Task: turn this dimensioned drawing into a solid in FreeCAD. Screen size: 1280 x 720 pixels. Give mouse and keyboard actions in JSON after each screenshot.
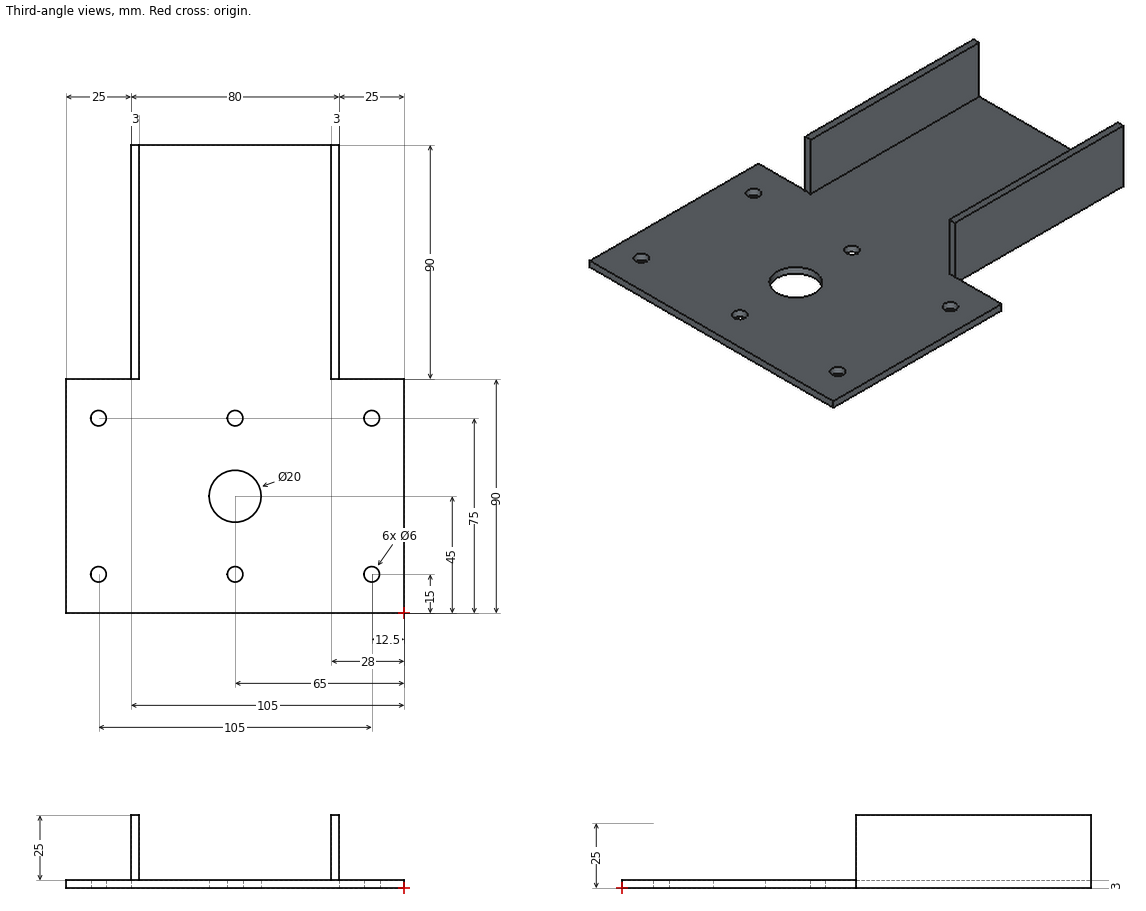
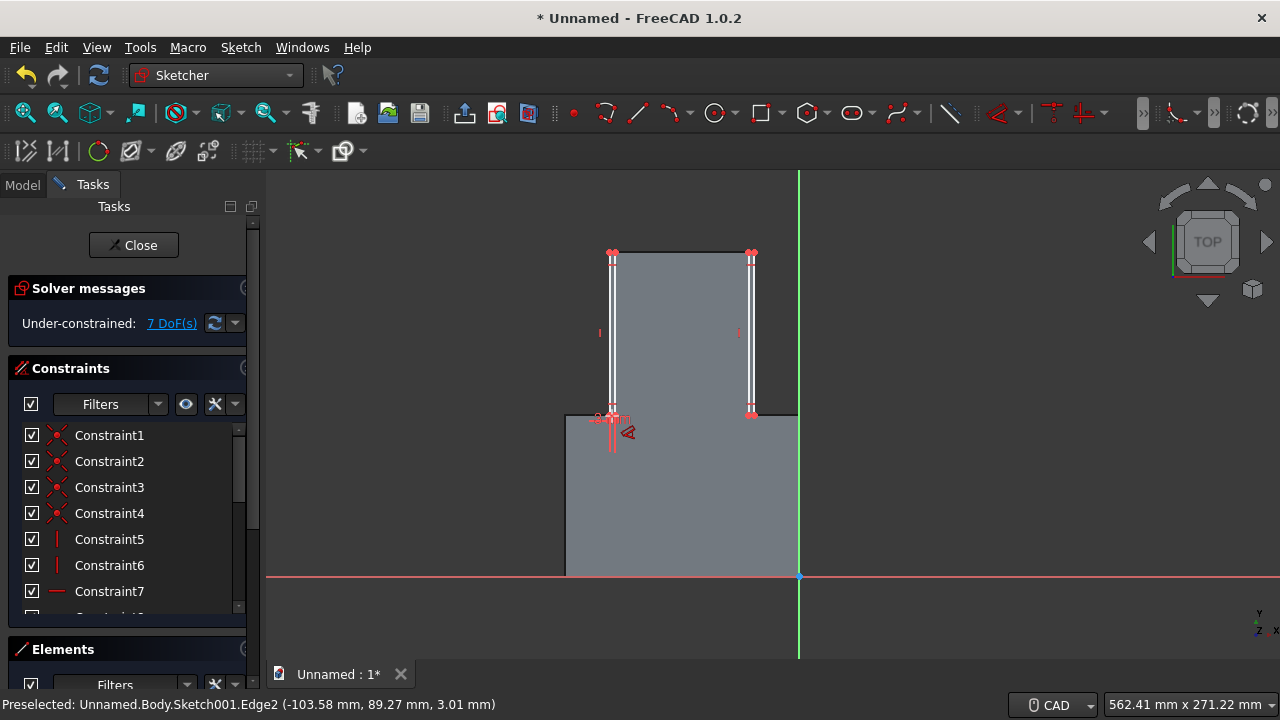
{"action": "scroll", "coordinate": [750, 416], "scroll_direction": "up", "scroll_amount": 11}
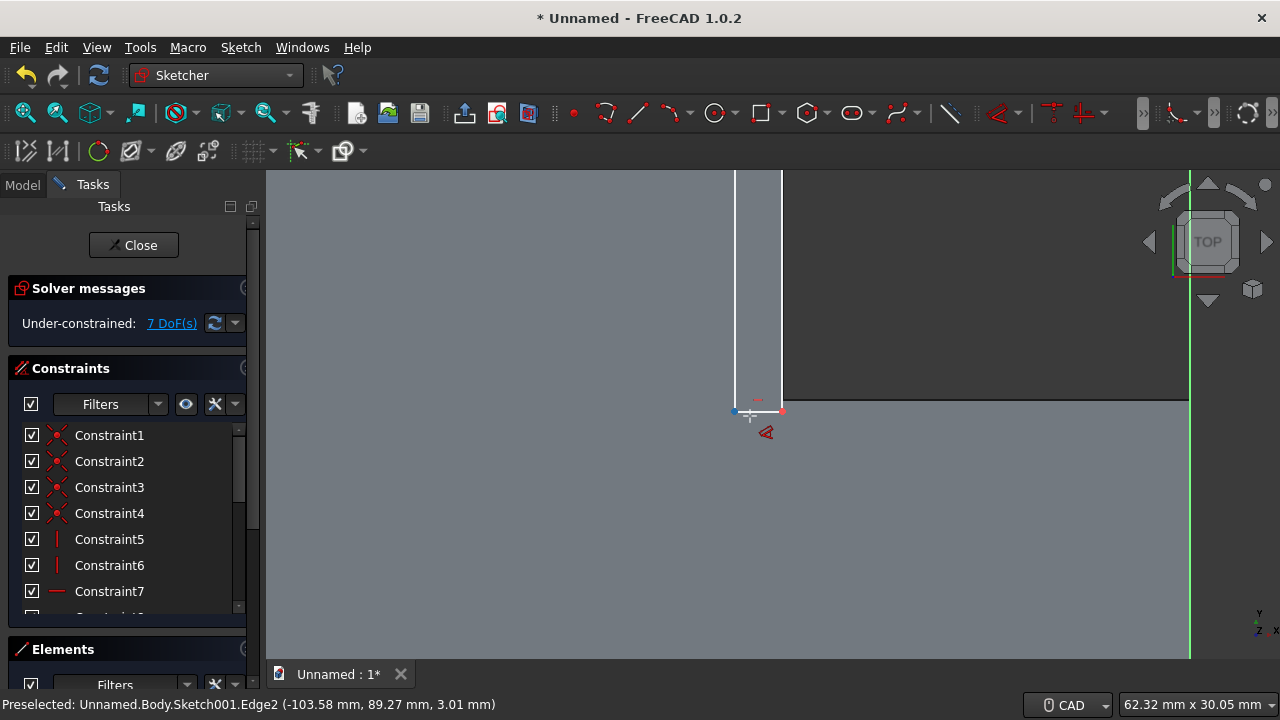
{"action": "left_click", "coordinate": [749, 412]}
{"action": "left_click", "coordinate": [758, 446]}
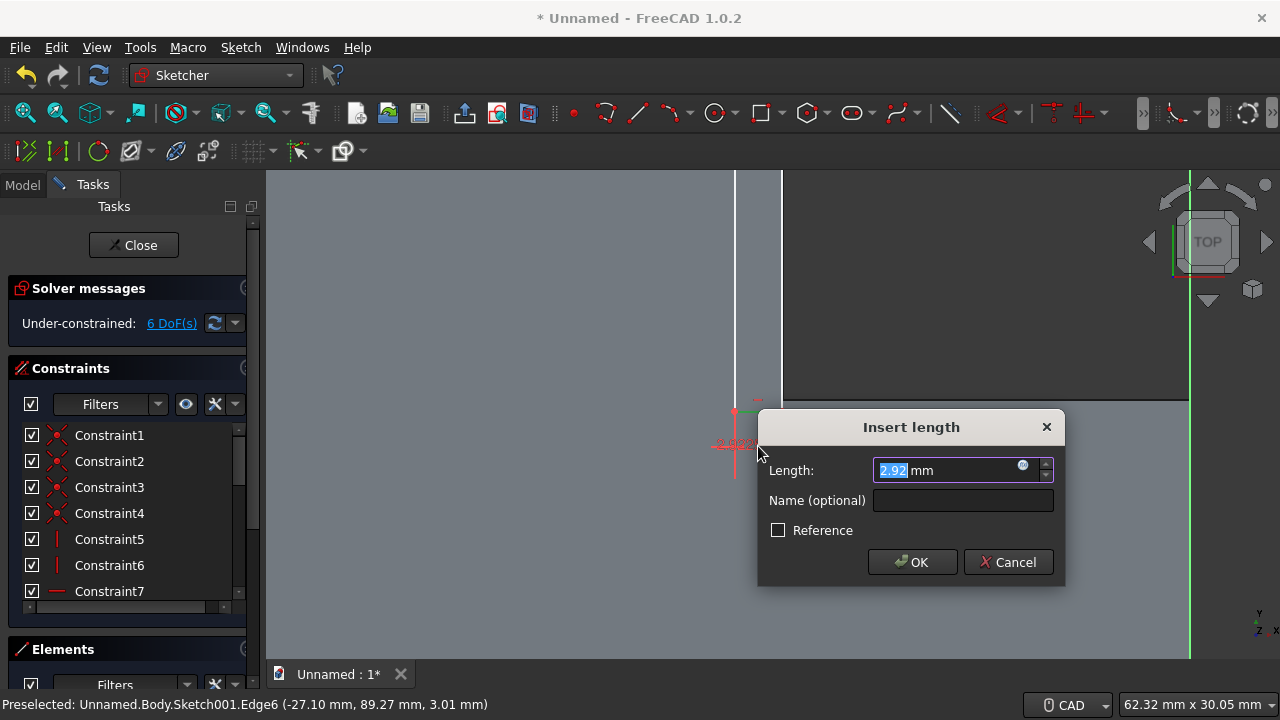
{"action": "type", "text": "3"}
{"action": "key", "text": "Return"}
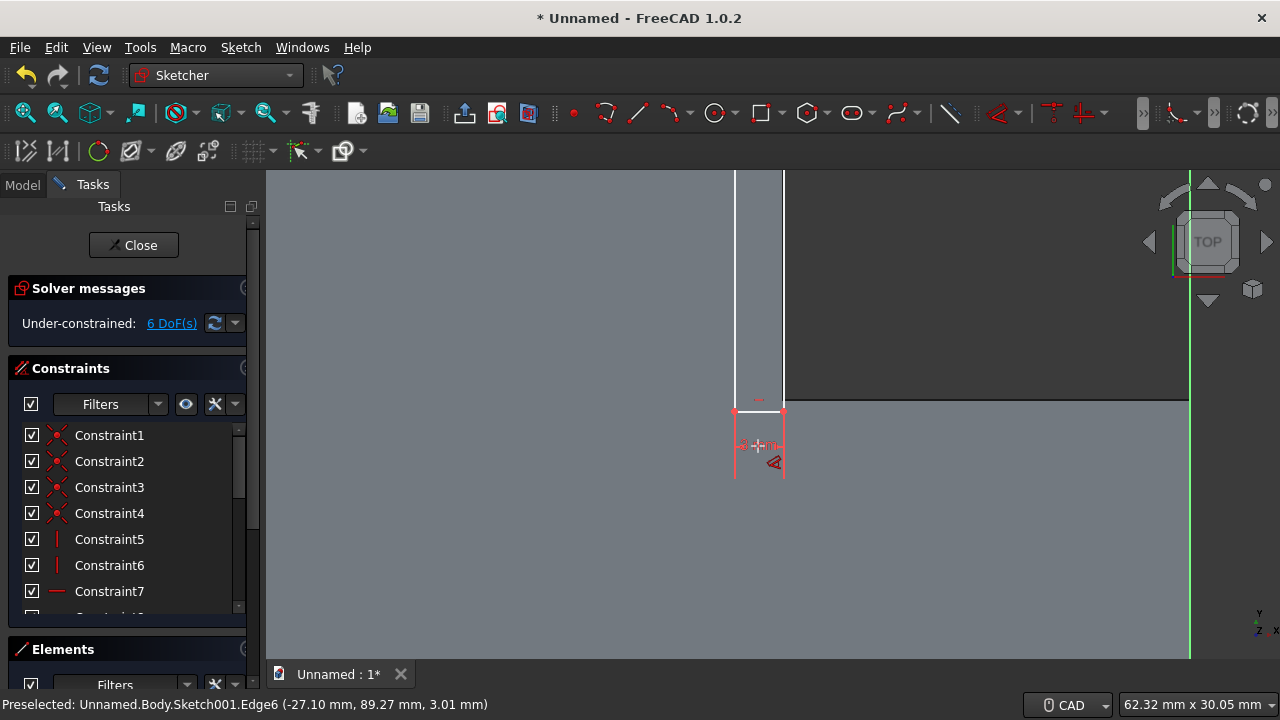
{"action": "scroll", "coordinate": [750, 416], "scroll_direction": "down", "scroll_amount": 11}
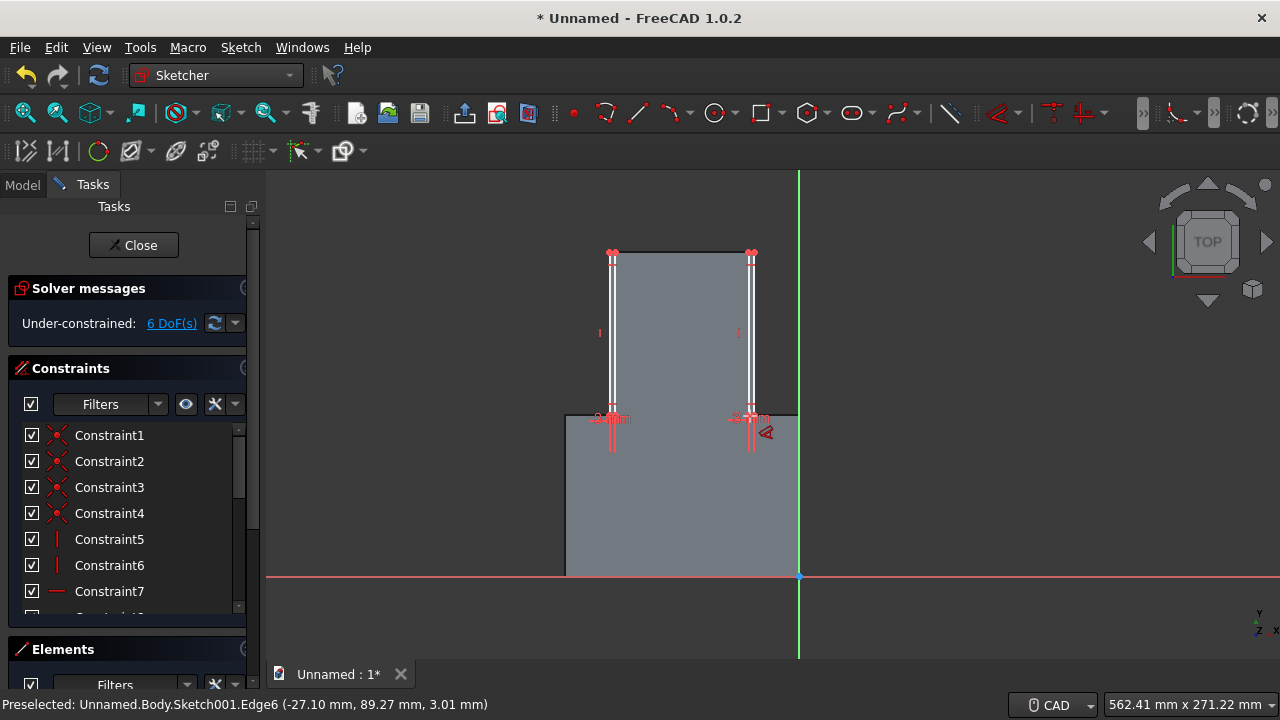
{"action": "scroll", "coordinate": [610, 302], "scroll_direction": "up", "scroll_amount": 5}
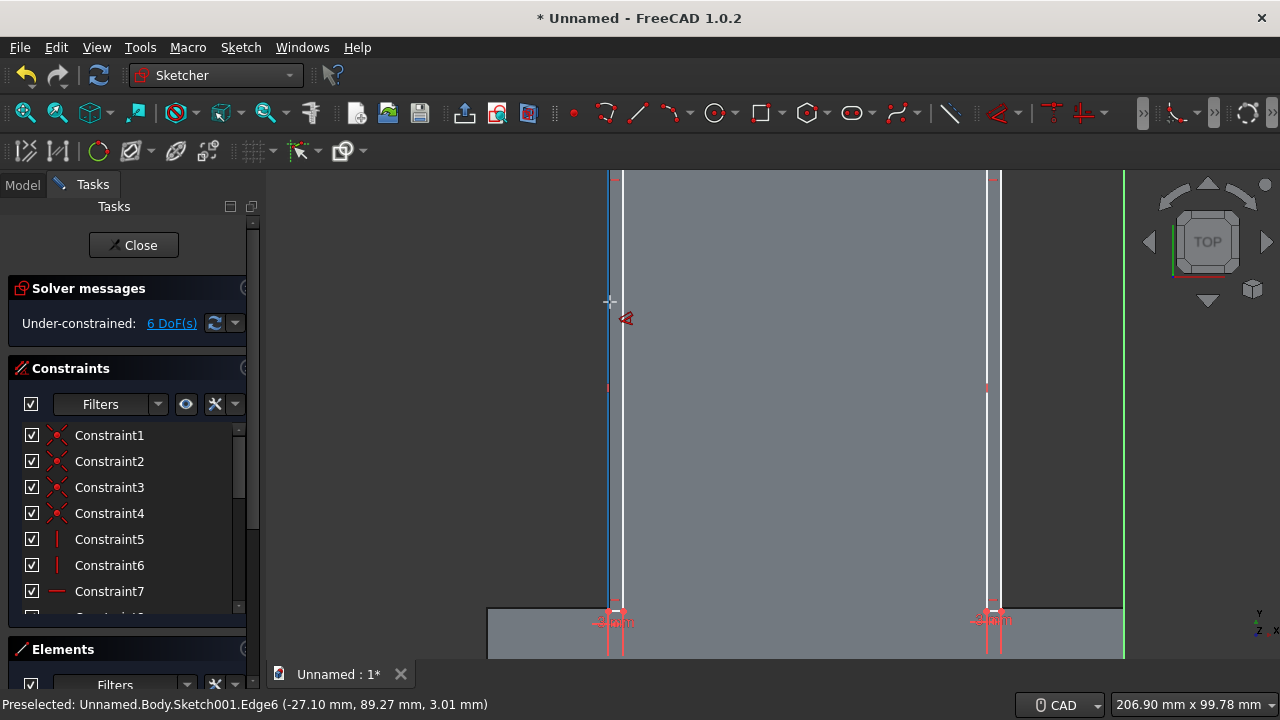
{"action": "left_click", "coordinate": [608, 301]}
{"action": "left_click", "coordinate": [574, 405]}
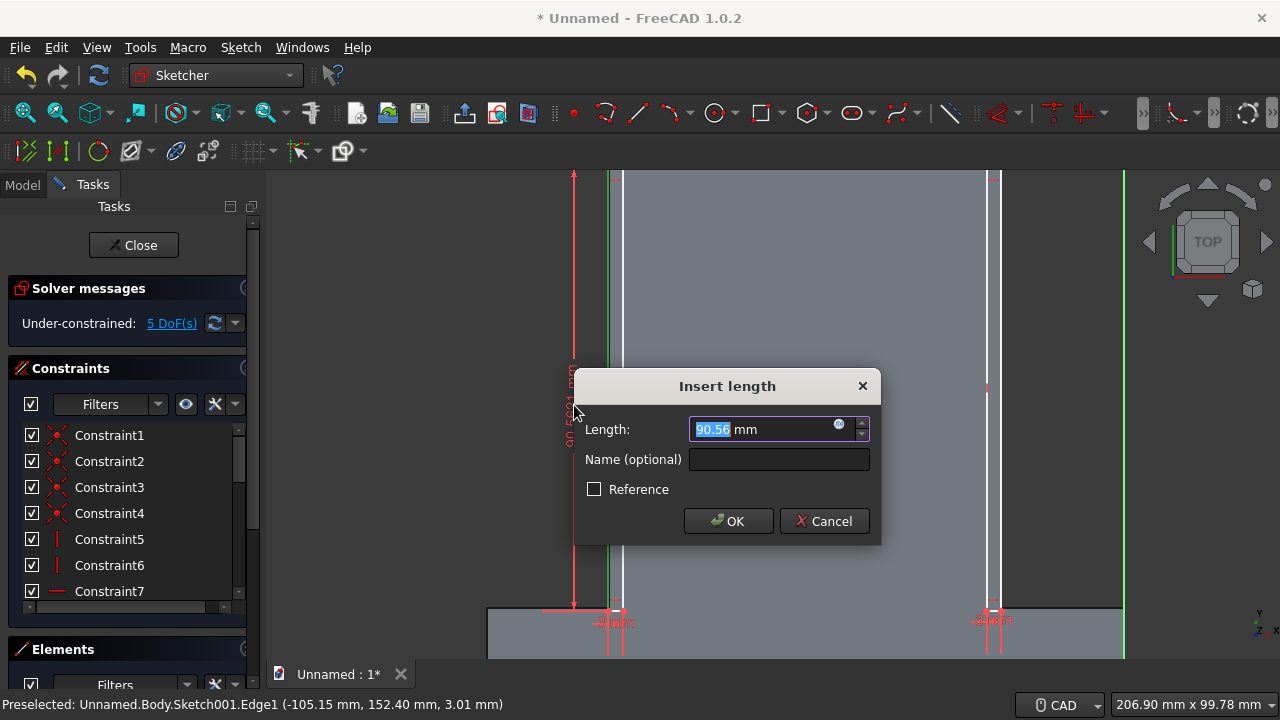
{"action": "type", "text": "90"}
{"action": "key", "text": "Return"}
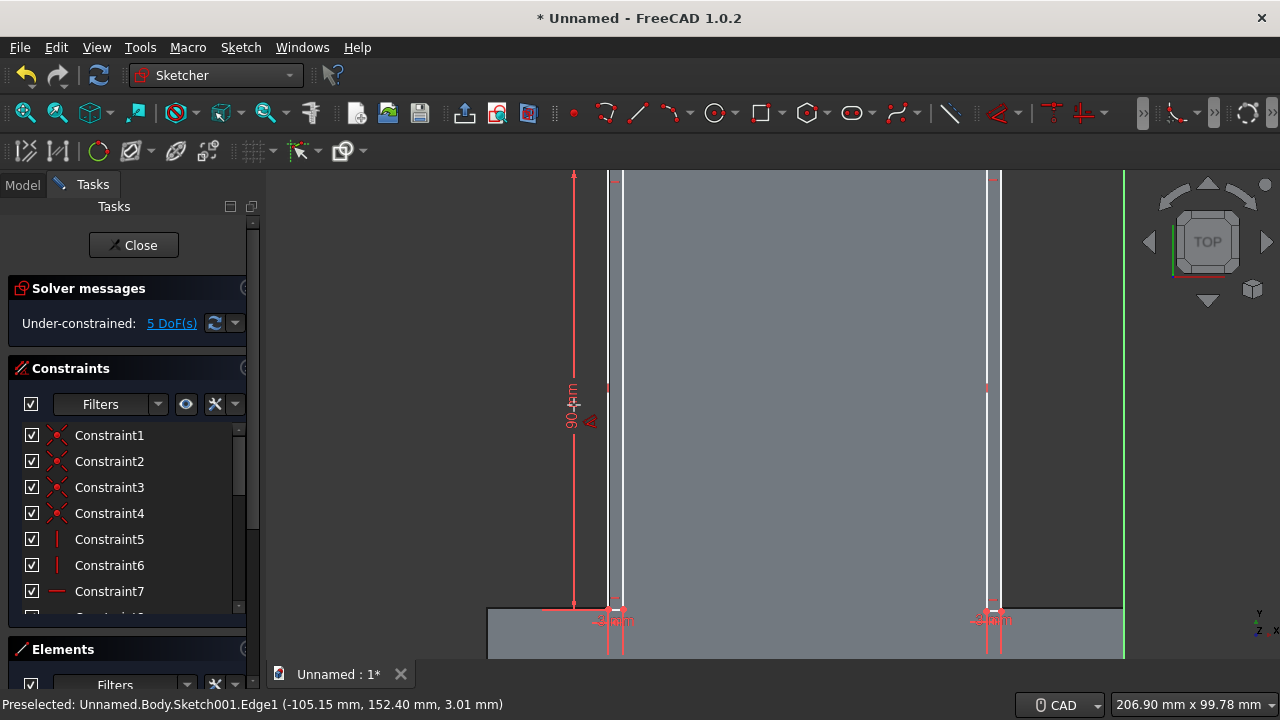
{"action": "left_click", "coordinate": [987, 301]}
{"action": "left_click", "coordinate": [1021, 405]}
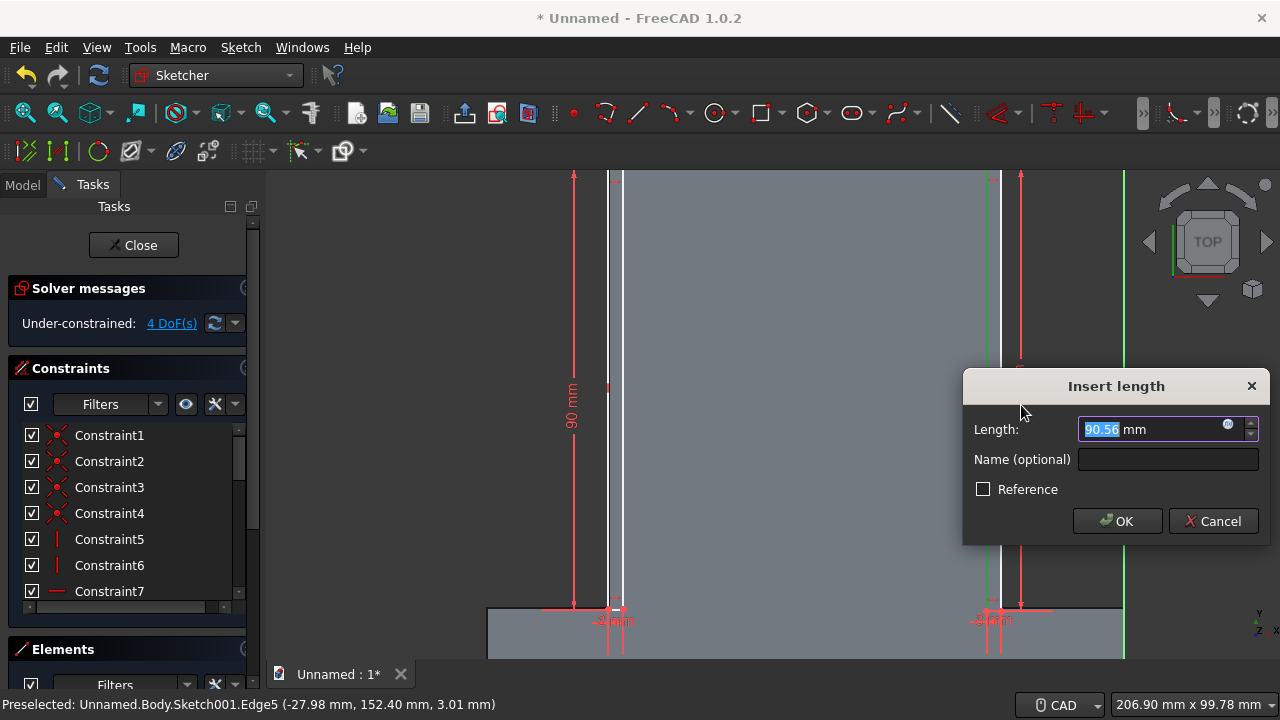
{"action": "type", "text": "90"}
{"action": "key", "text": "Return"}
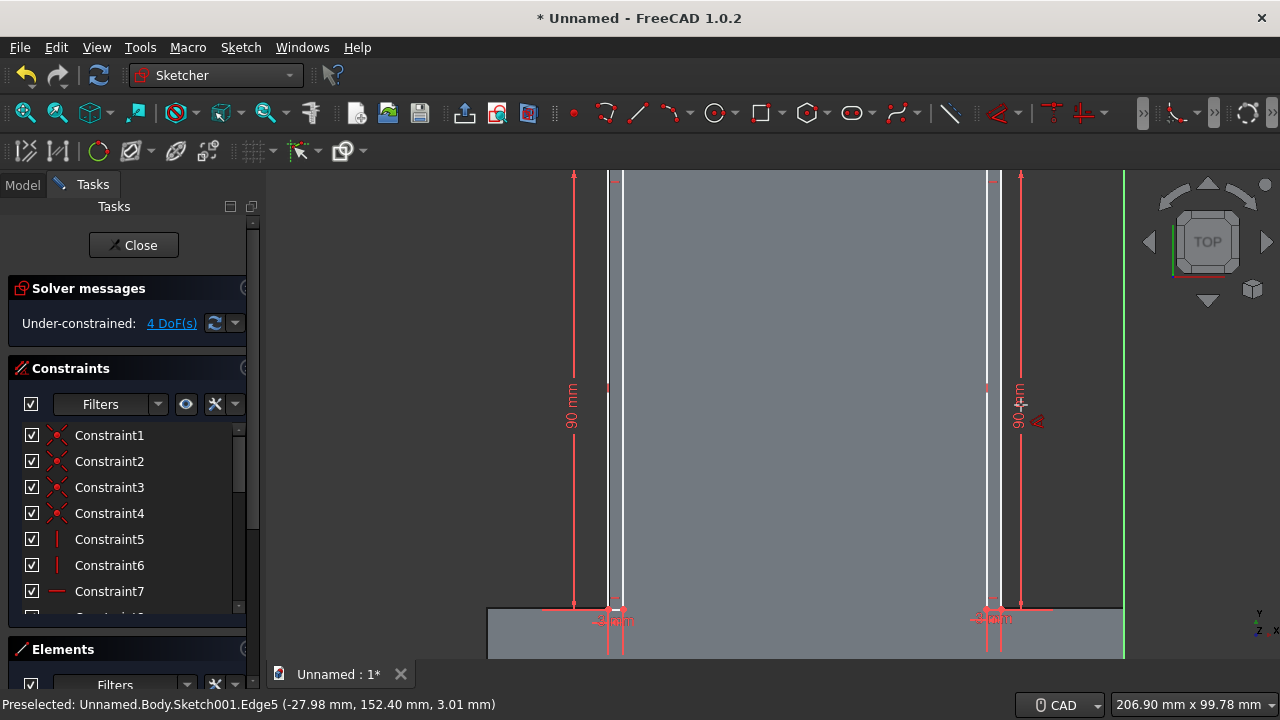
{"action": "left_click", "coordinate": [608, 610]}
{"action": "left_click", "coordinate": [526, 620]}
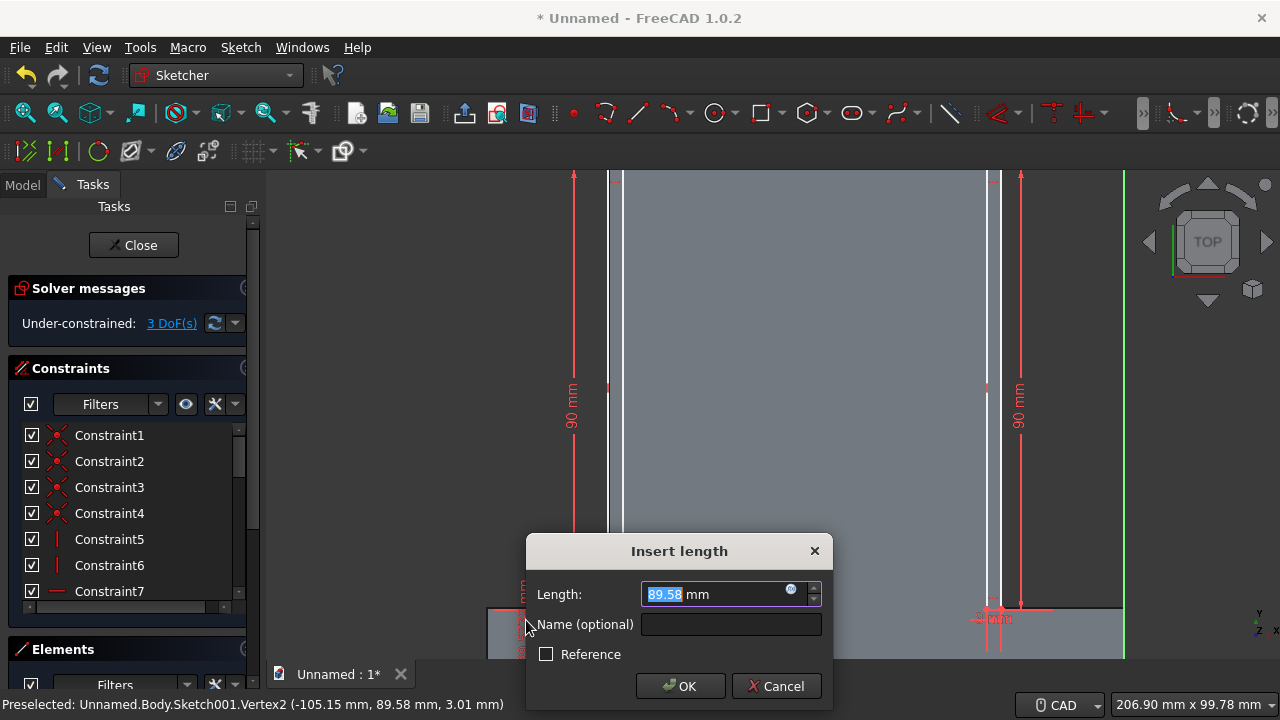
{"action": "type", "text": "90"}
{"action": "key", "text": "Return"}